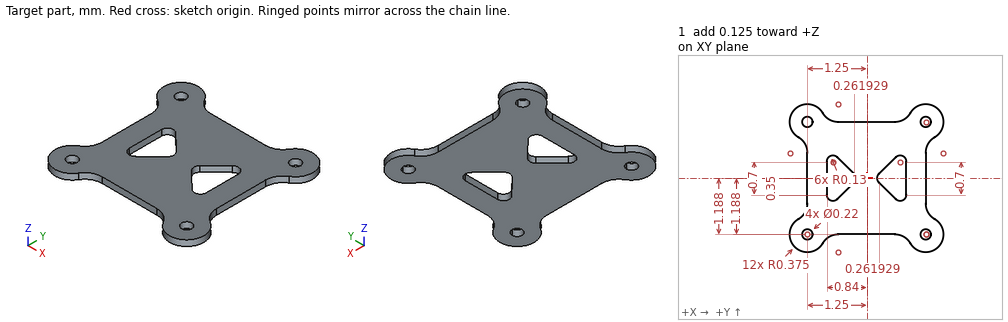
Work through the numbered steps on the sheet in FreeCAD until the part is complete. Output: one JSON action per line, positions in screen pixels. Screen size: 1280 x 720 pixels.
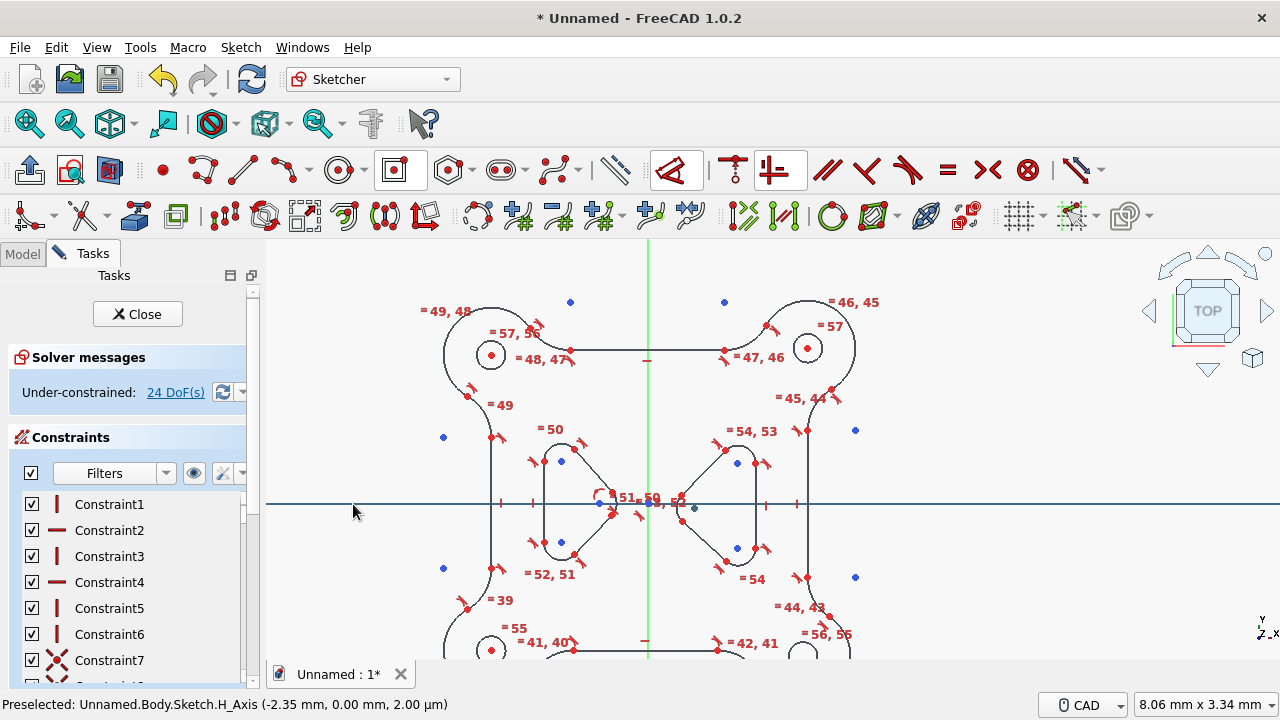
{"action": "left_click", "coordinate": [734, 170]}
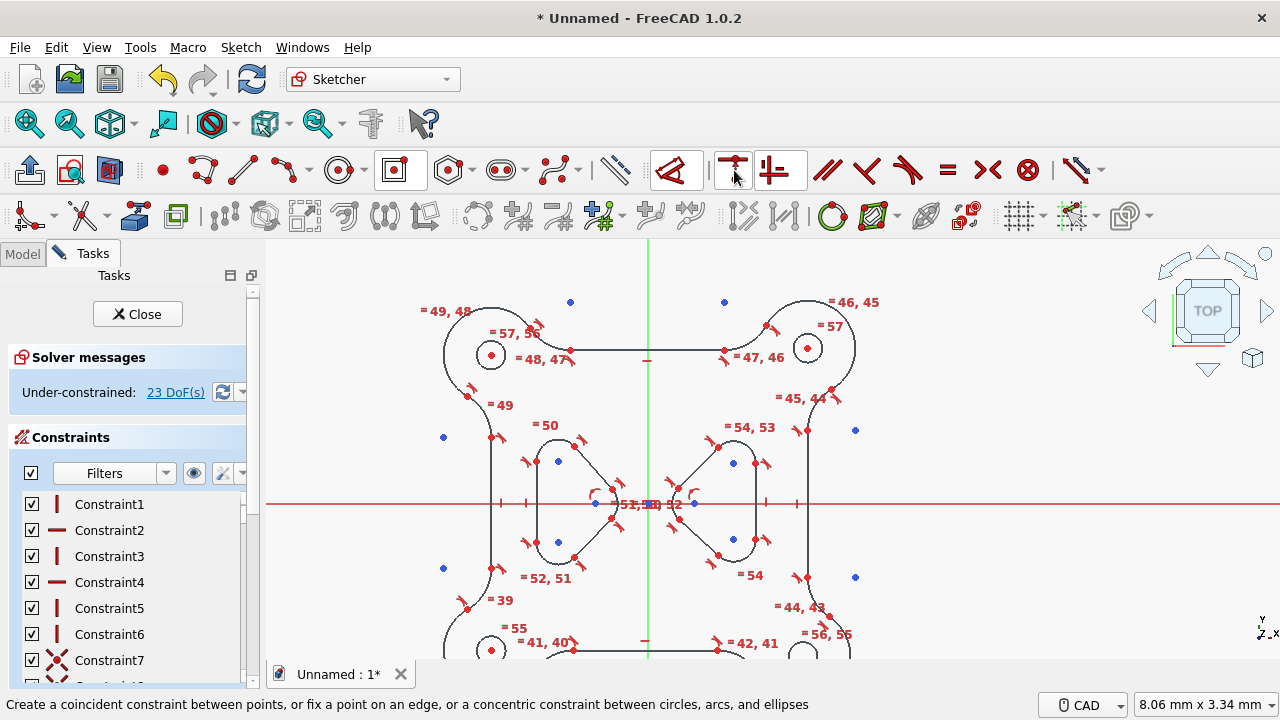
{"action": "scroll", "coordinate": [818, 338], "scroll_direction": "down", "scroll_amount": 2}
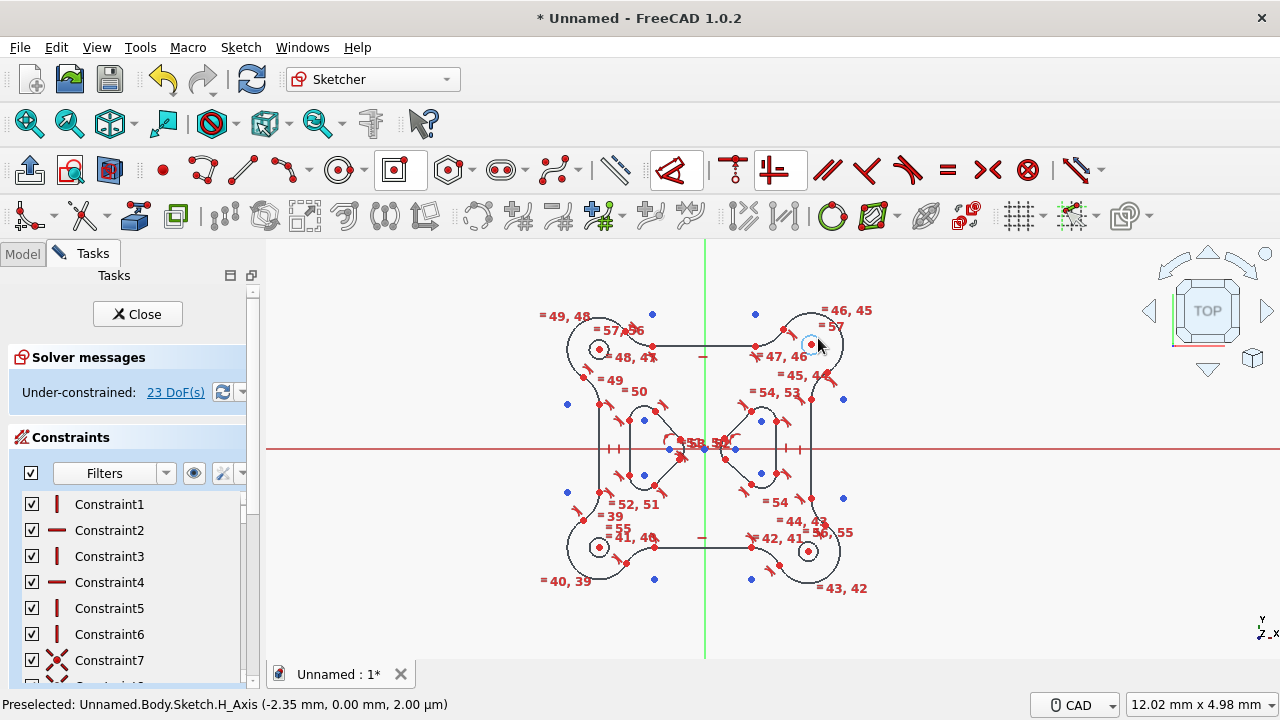
{"action": "left_click", "coordinate": [599, 548]}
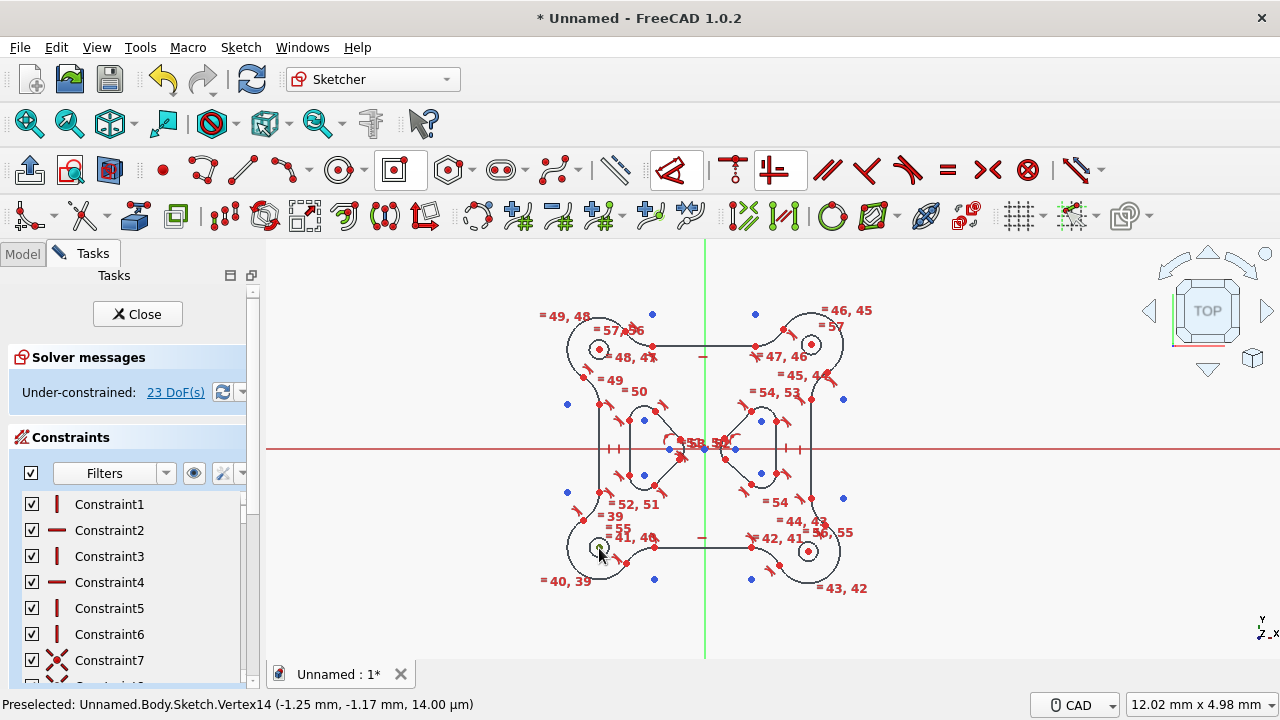
{"action": "left_click", "coordinate": [808, 552]}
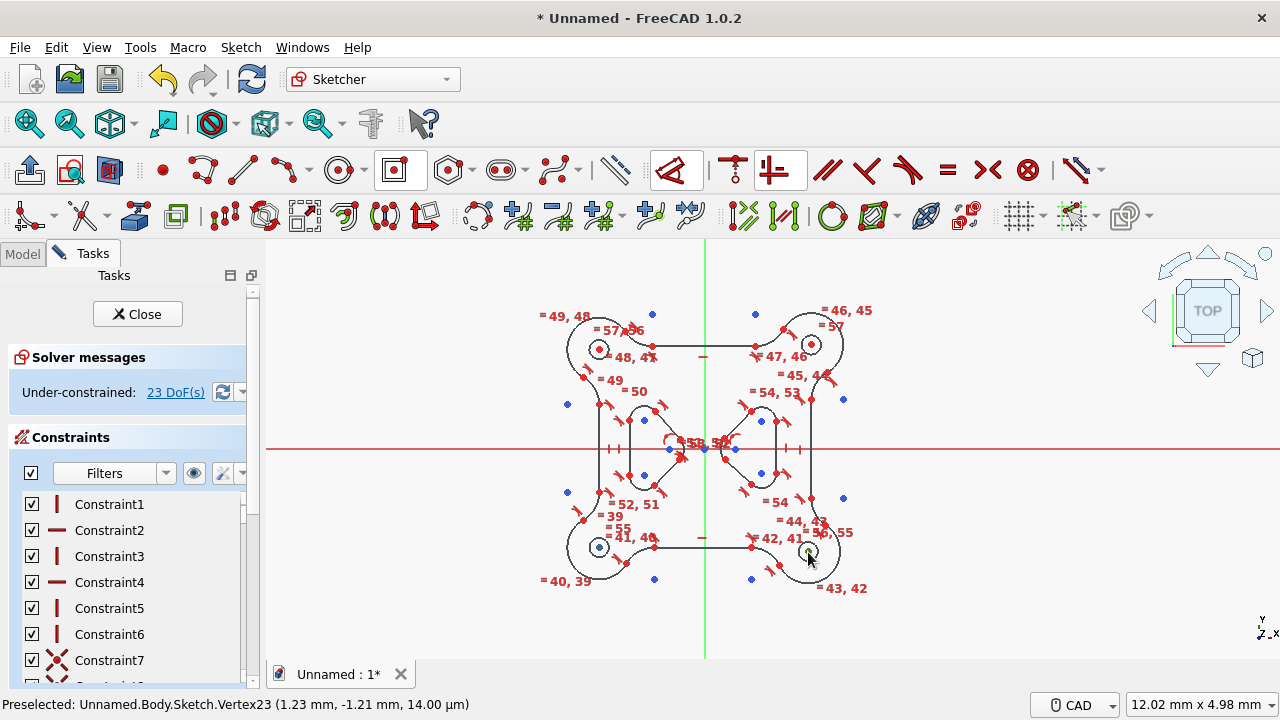
{"action": "left_click", "coordinate": [705, 605]}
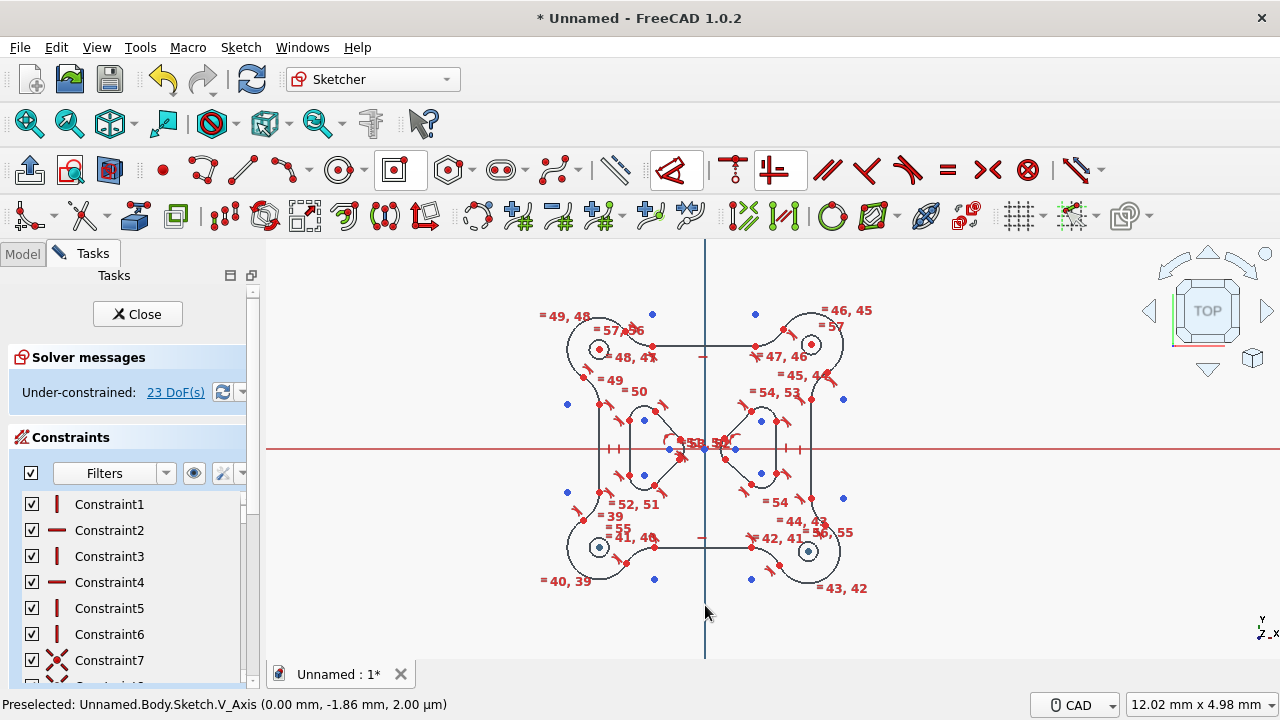
{"action": "left_click", "coordinate": [988, 170]}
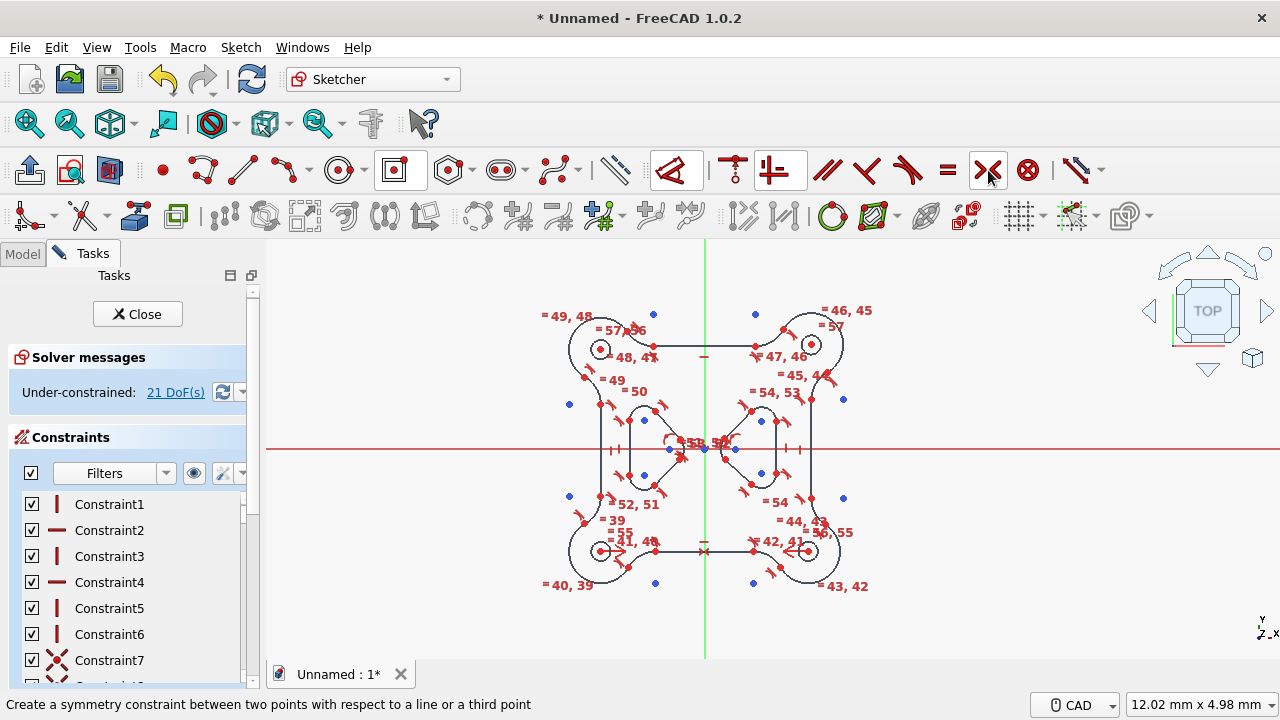
{"action": "left_click", "coordinate": [808, 551]}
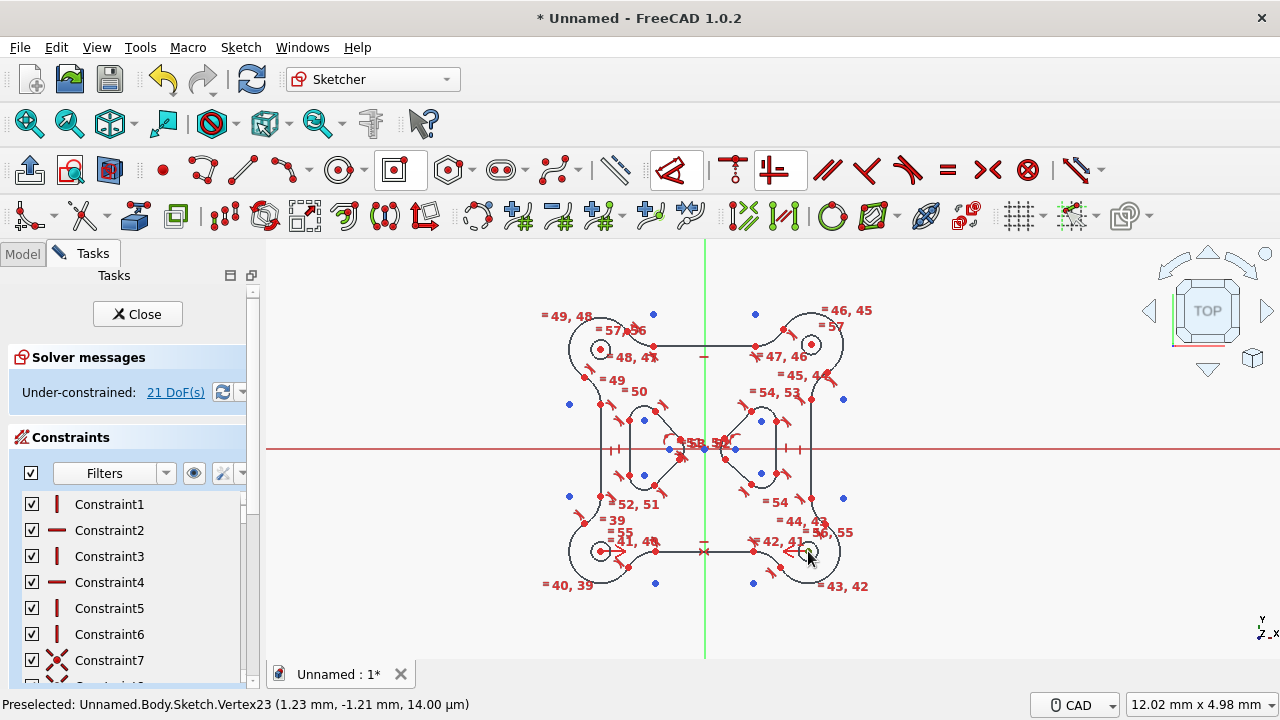
{"action": "left_click", "coordinate": [811, 345]}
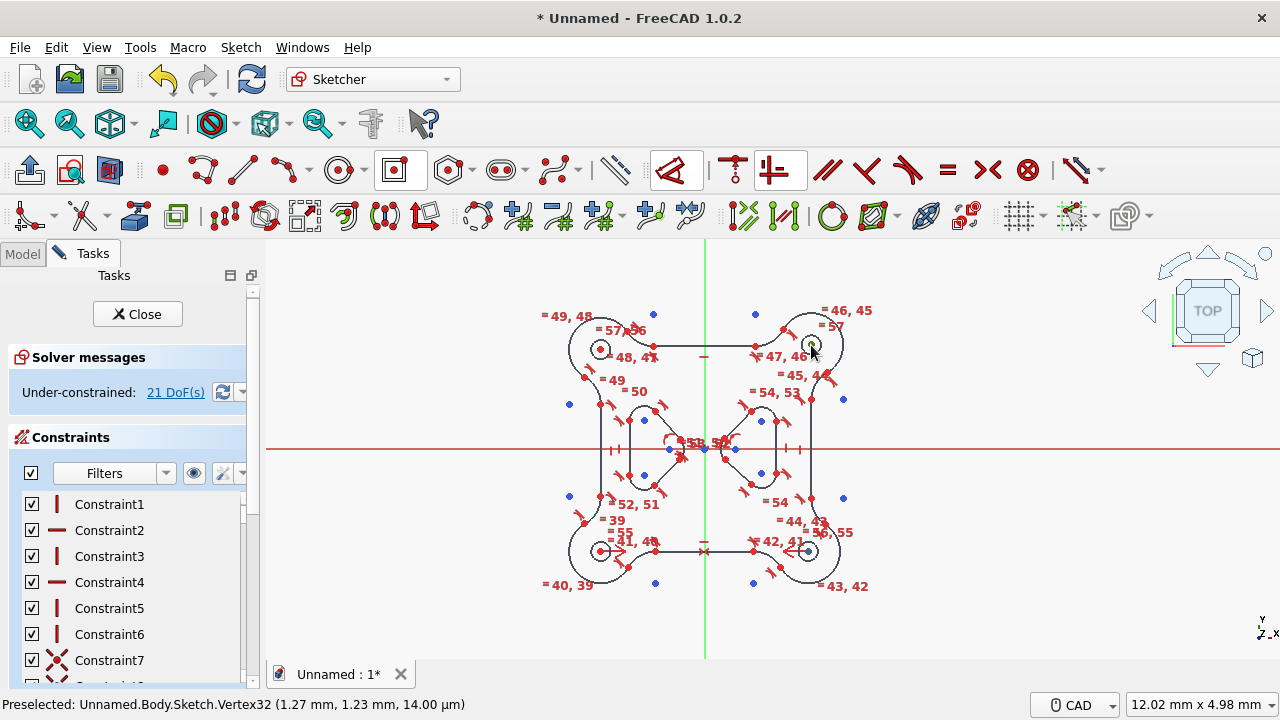
{"action": "left_click", "coordinate": [353, 449]}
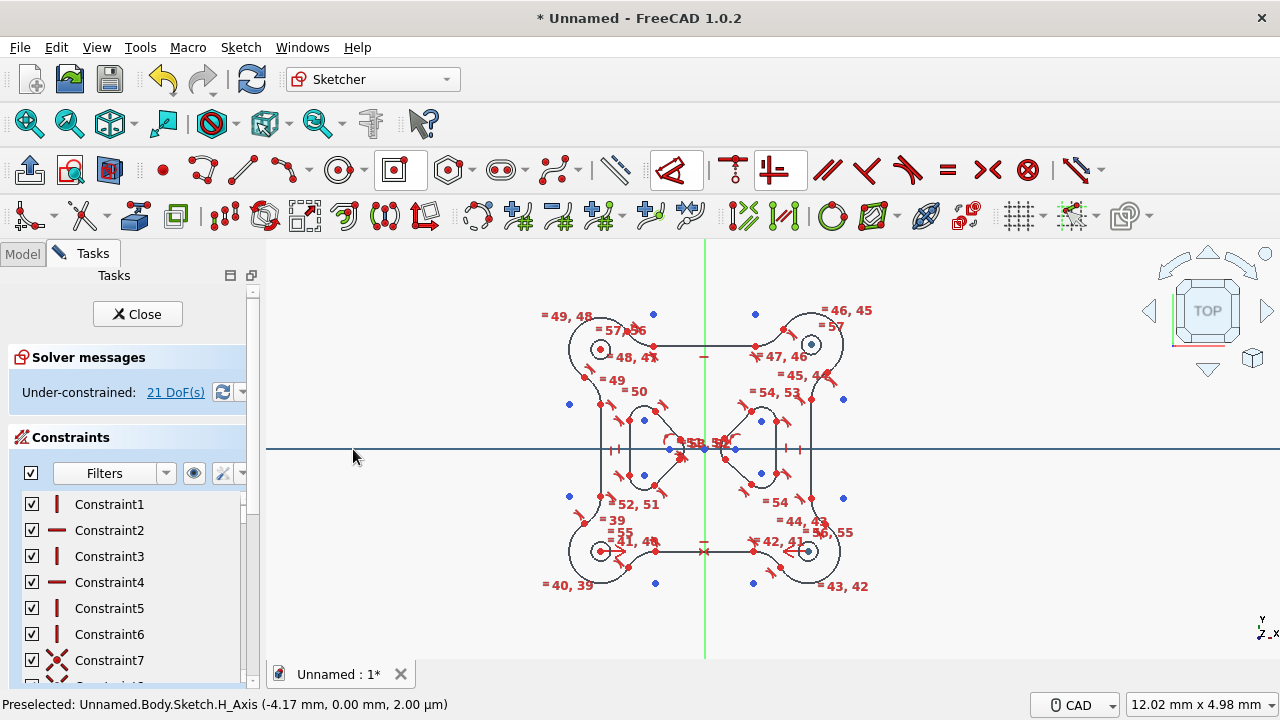
{"action": "left_click", "coordinate": [988, 170]}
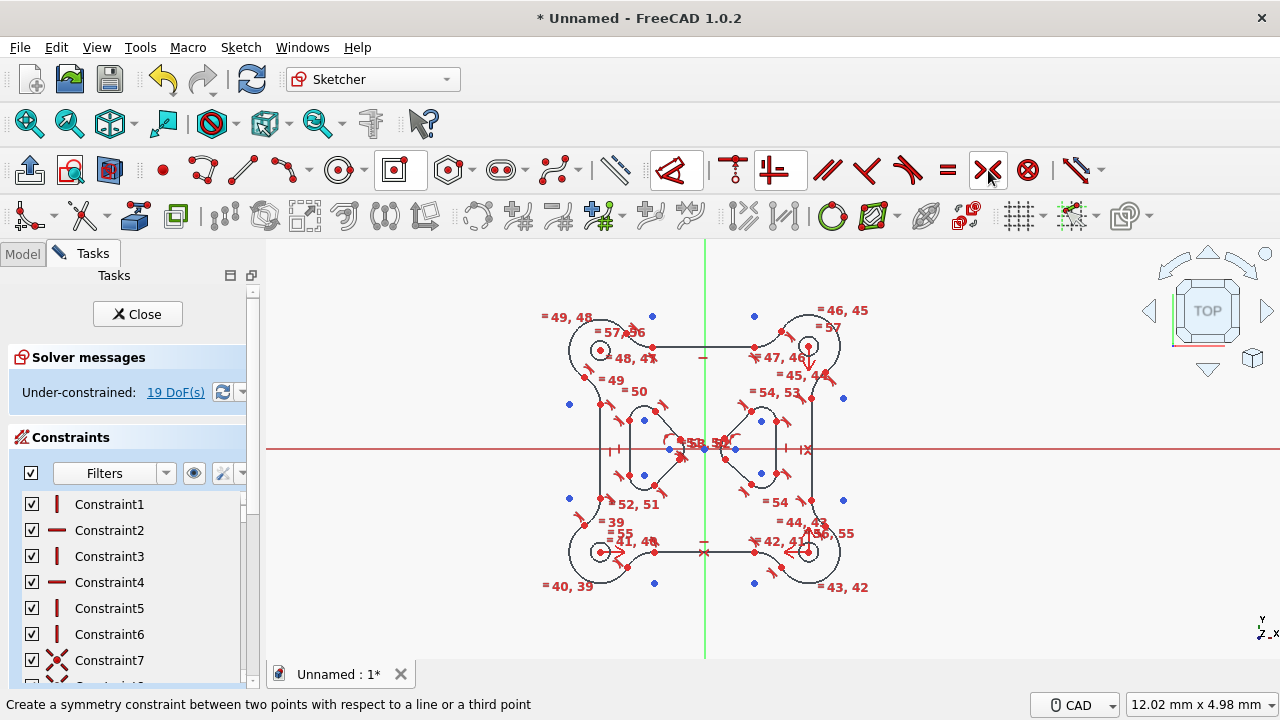
{"action": "left_click", "coordinate": [654, 583]}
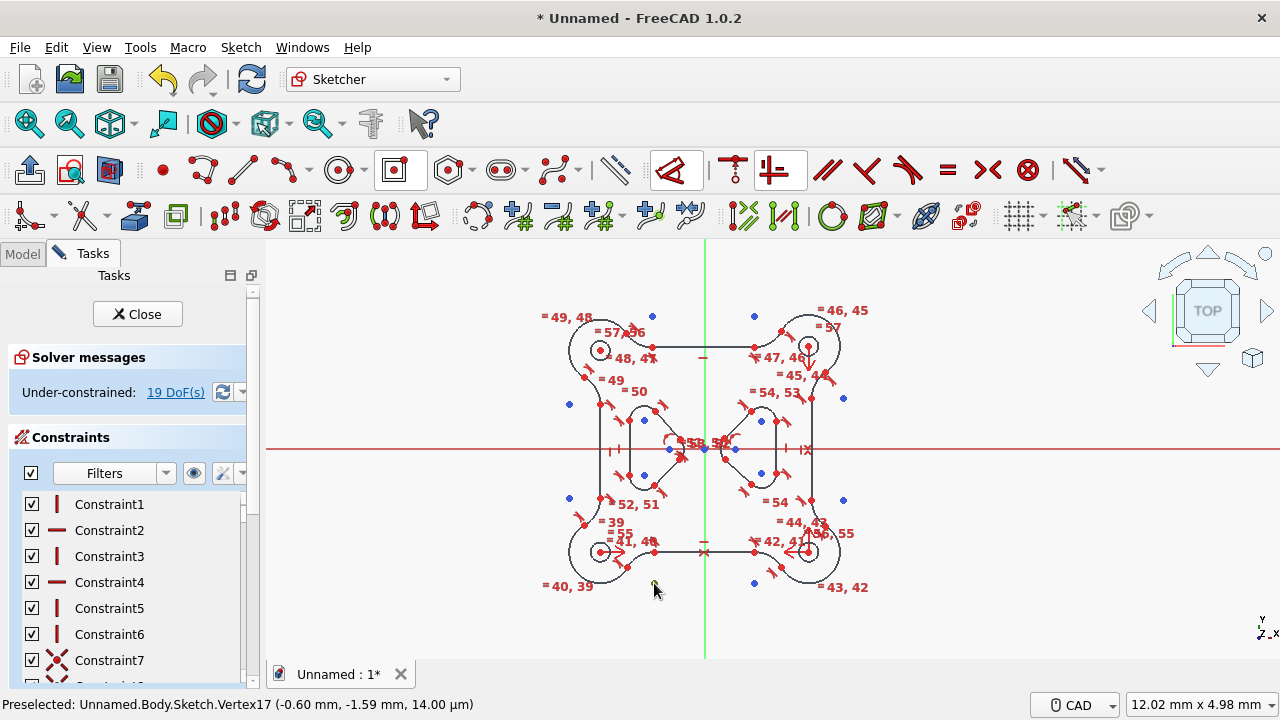
{"action": "left_click", "coordinate": [652, 316]}